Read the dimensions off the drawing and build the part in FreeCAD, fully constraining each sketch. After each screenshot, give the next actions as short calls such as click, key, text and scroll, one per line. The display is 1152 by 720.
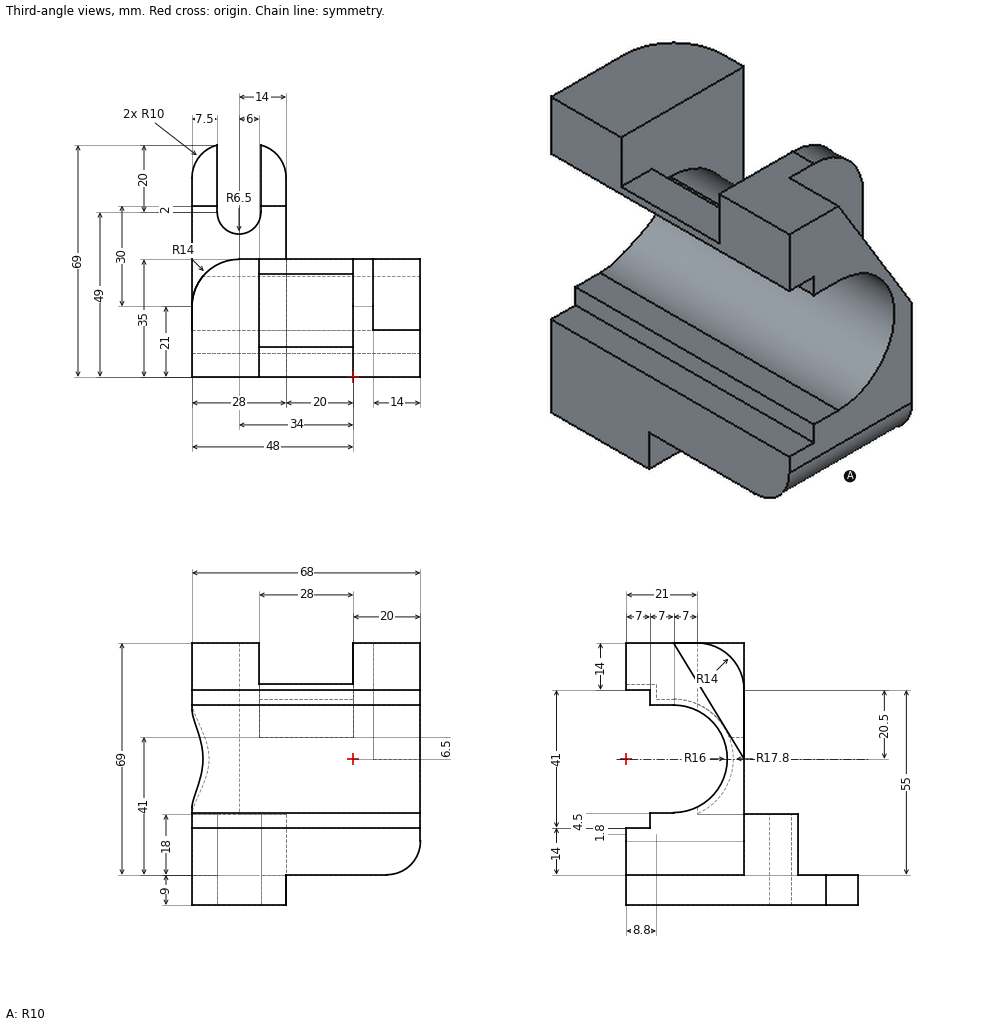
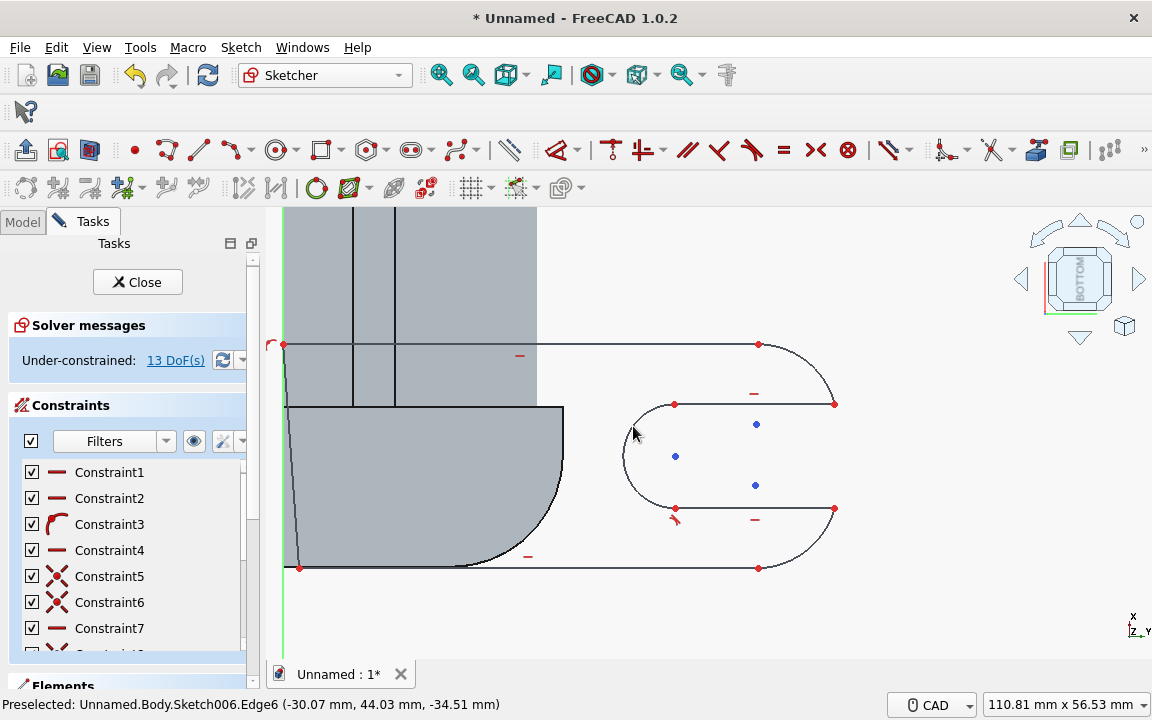
click(723, 404)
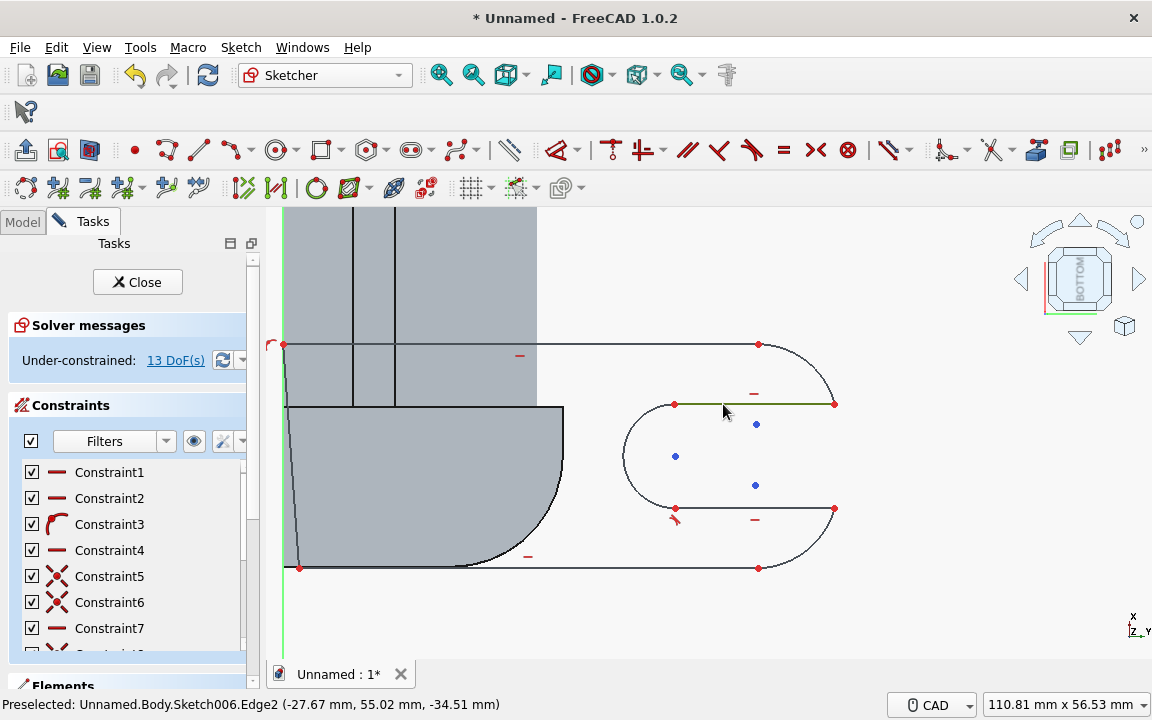
click(633, 426)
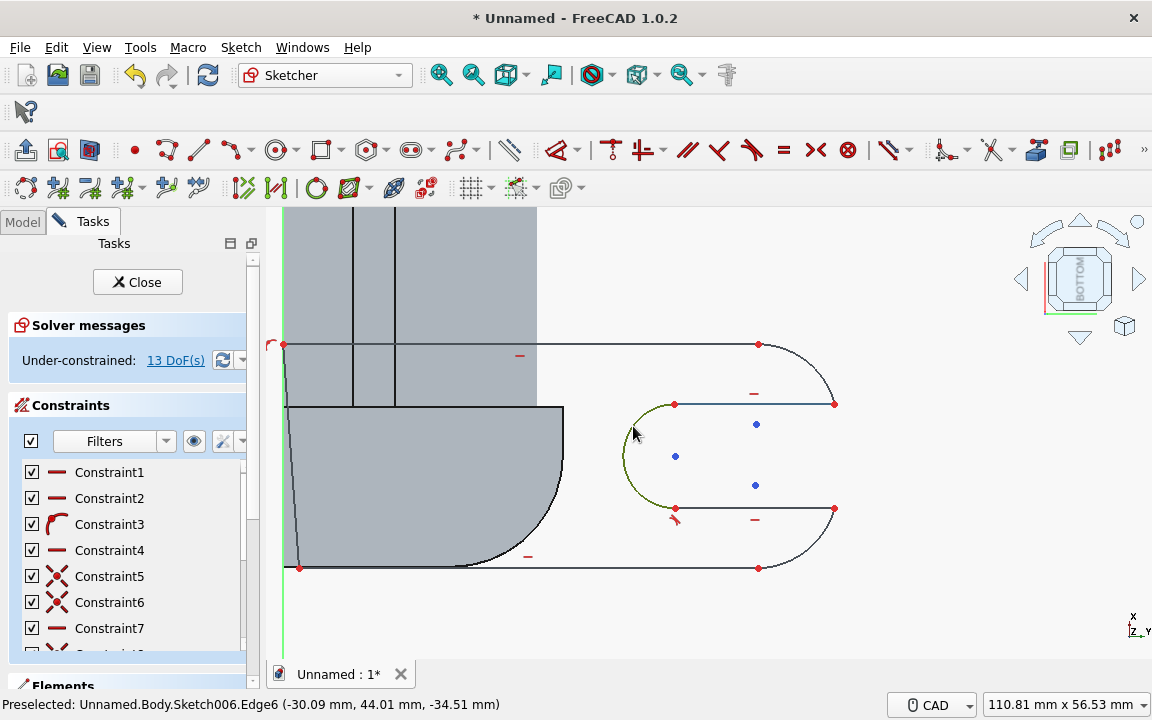
click(752, 150)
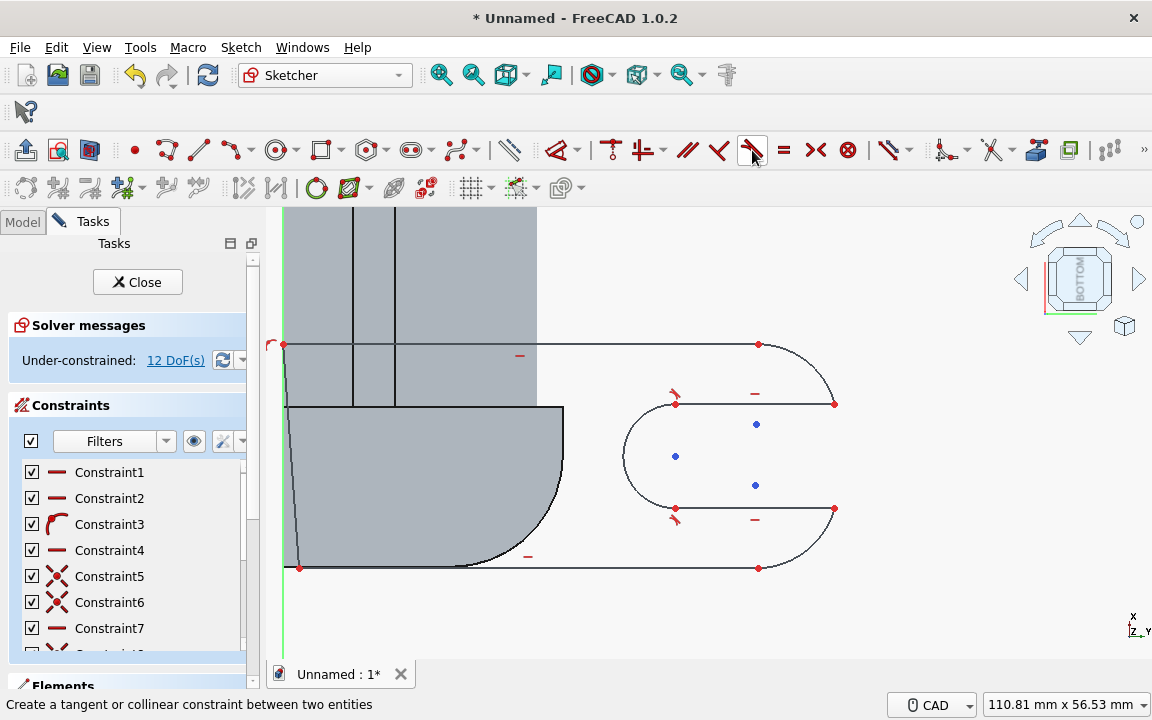
click(616, 344)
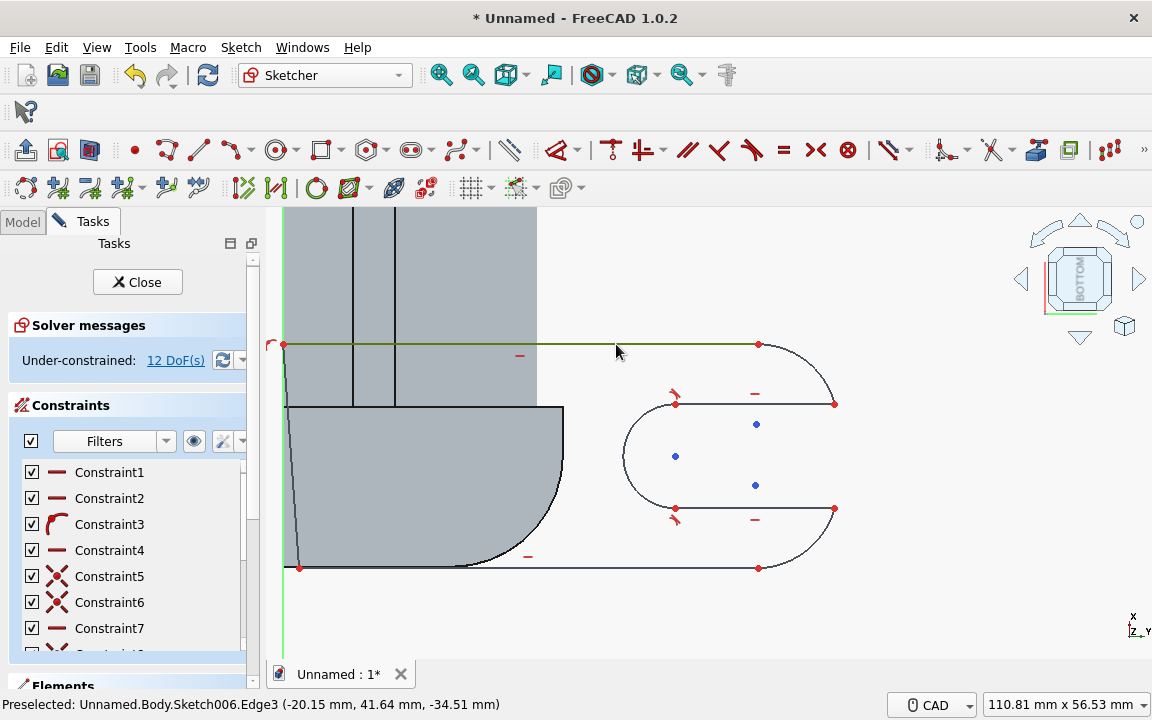
click(821, 376)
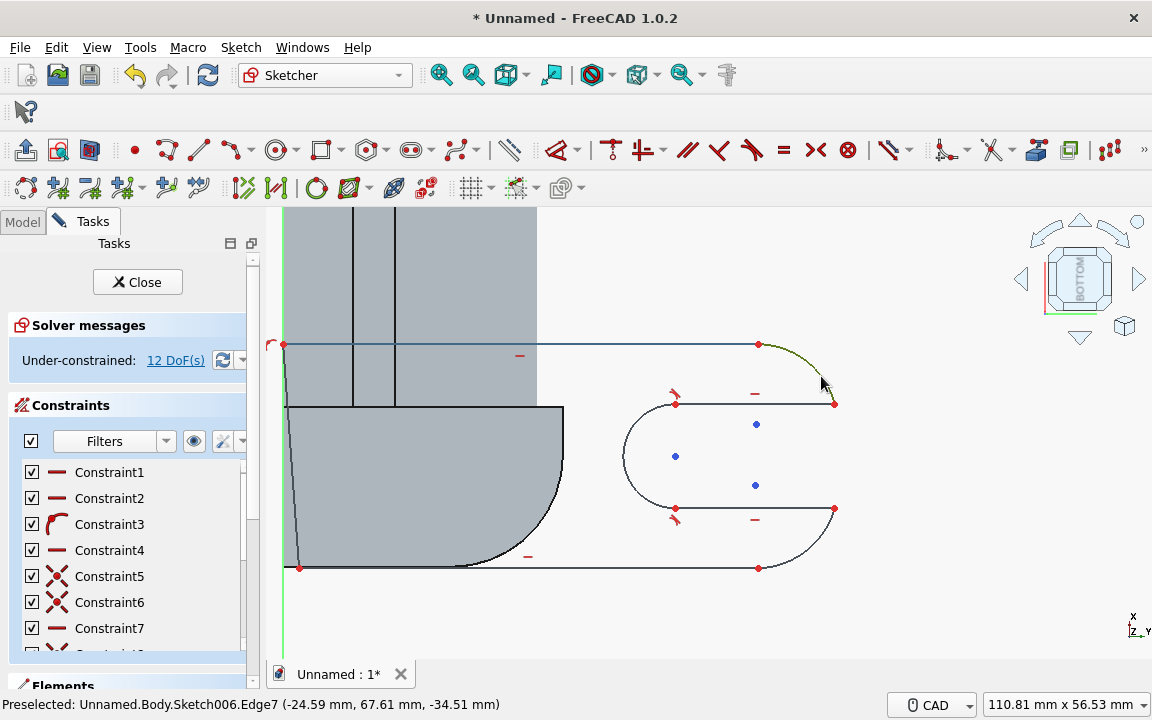
click(752, 150)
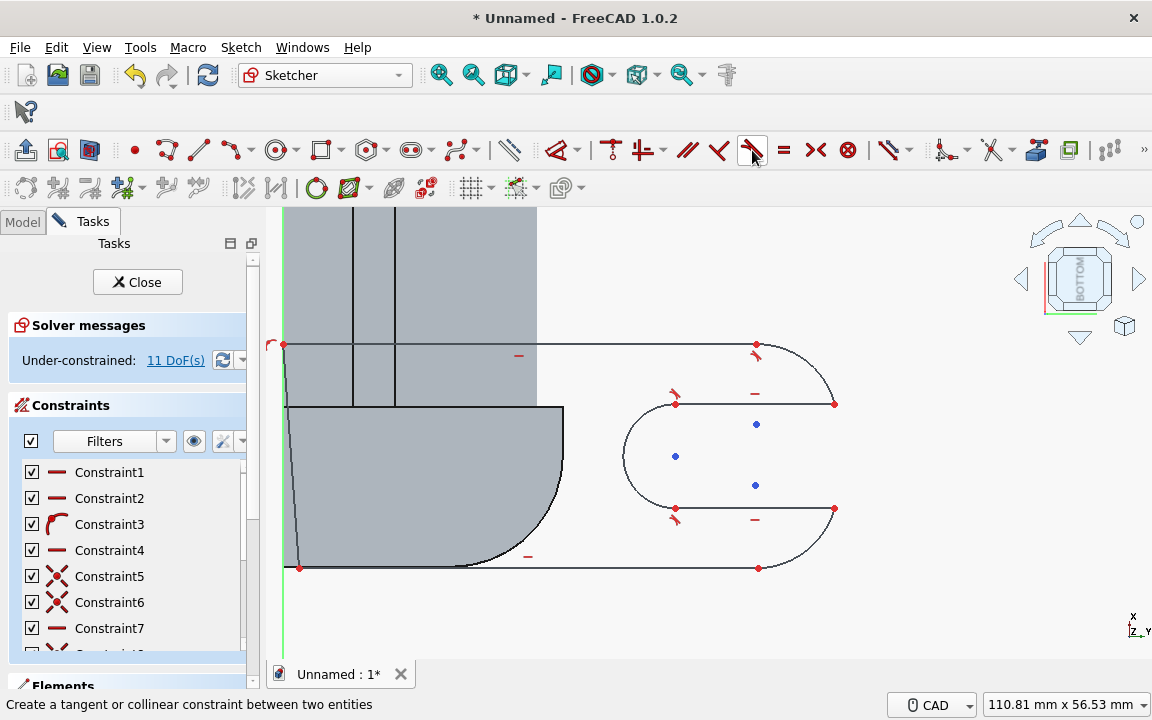
click(437, 568)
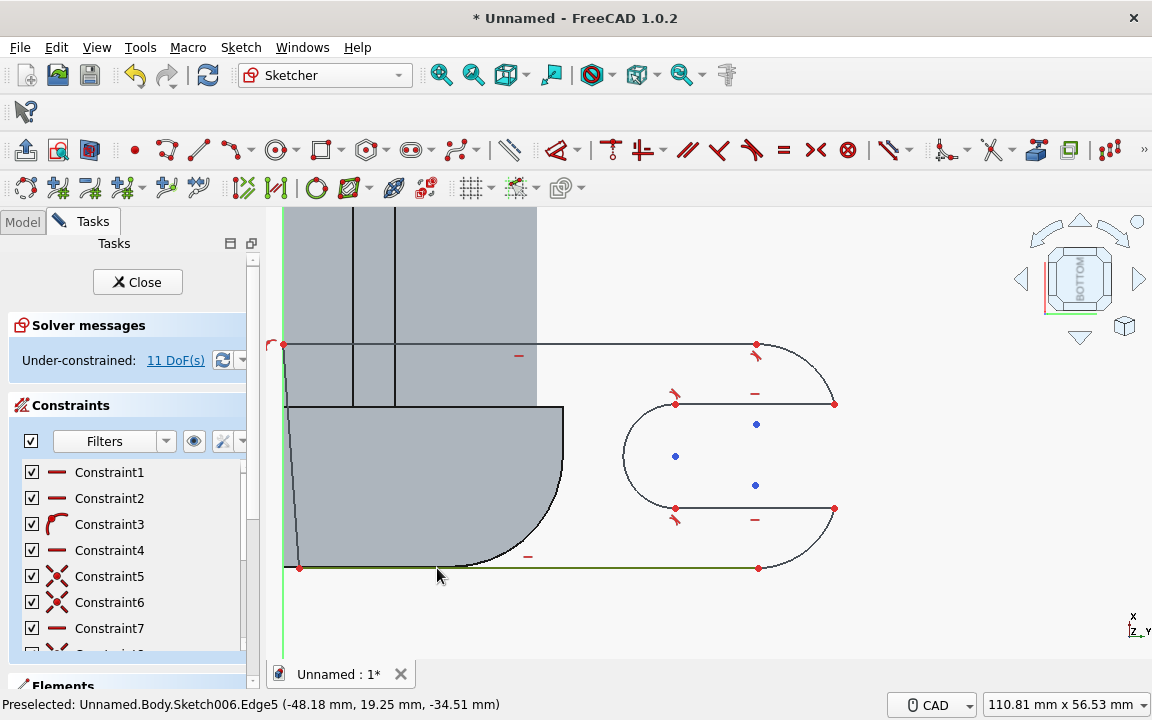
click(789, 561)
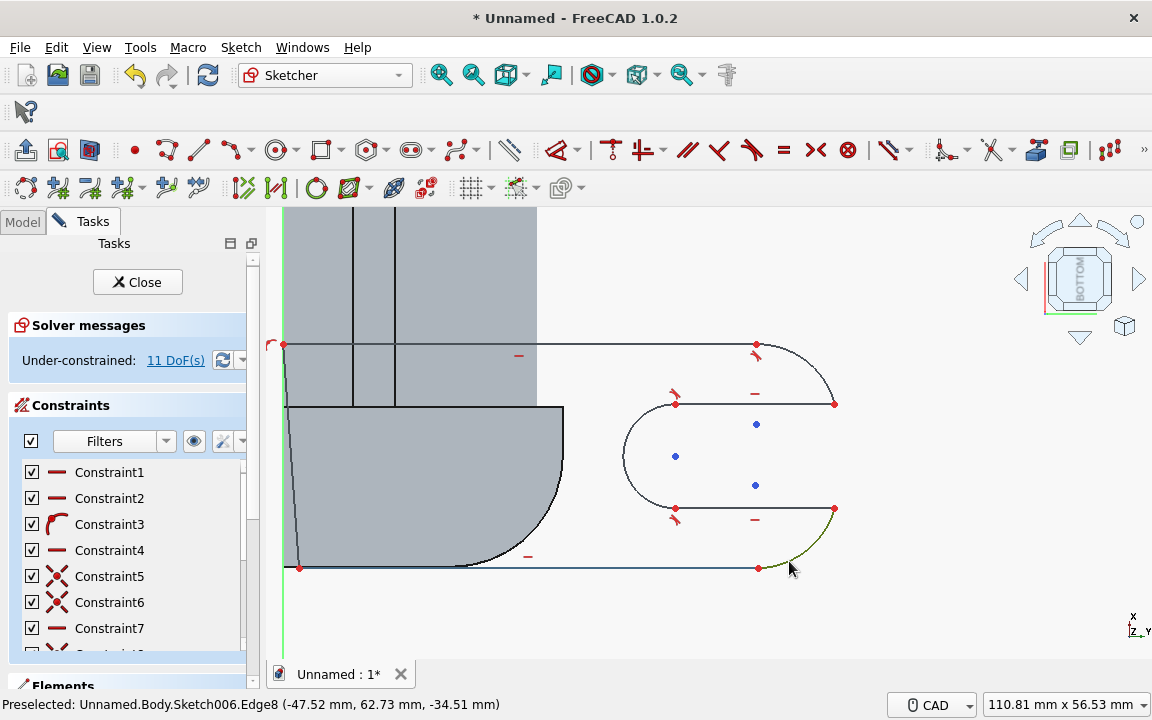
key(t)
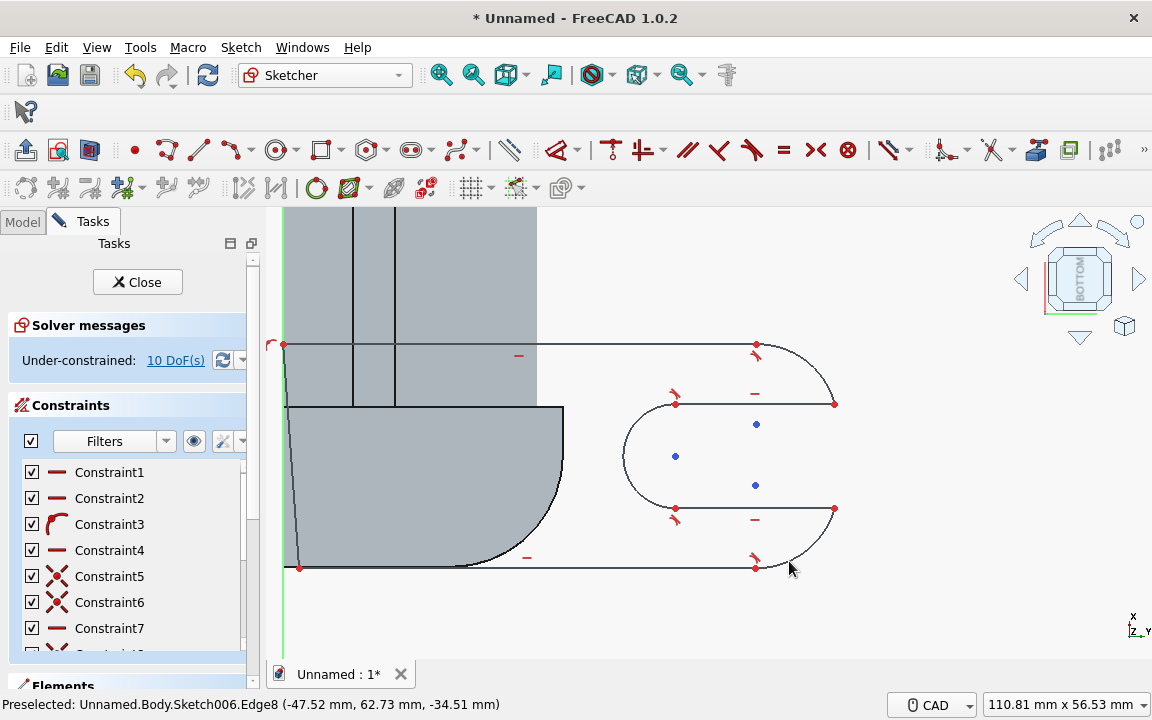
scroll(294, 501, up, 2)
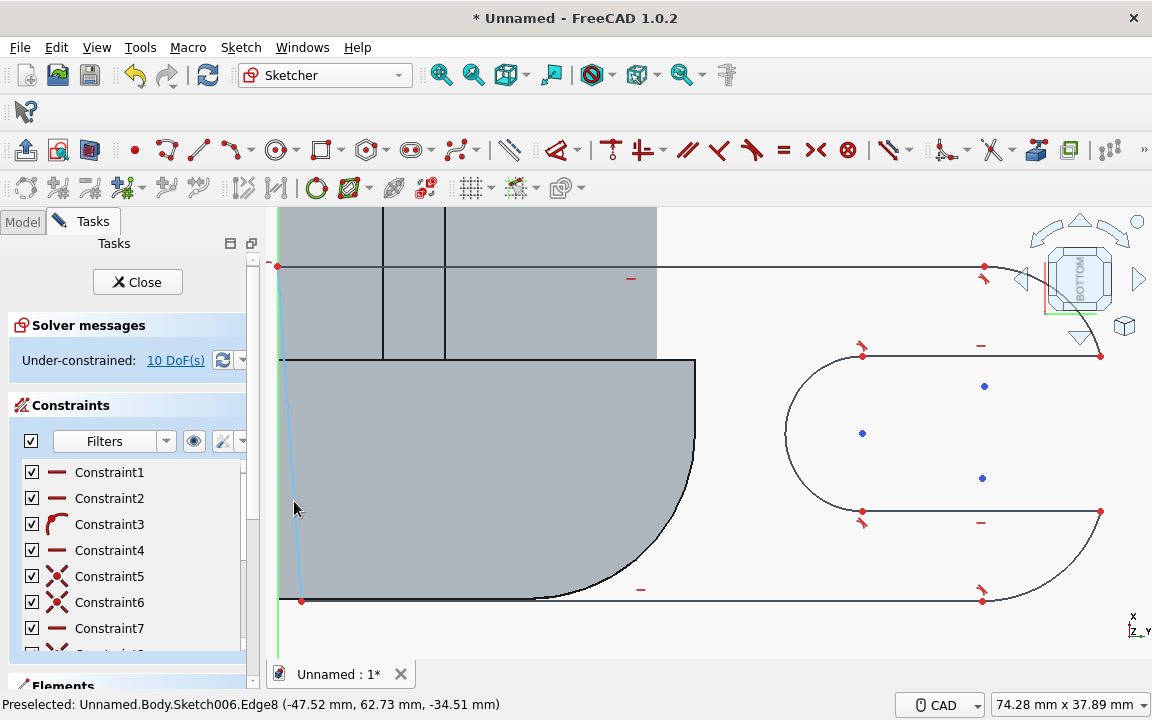
click(294, 501)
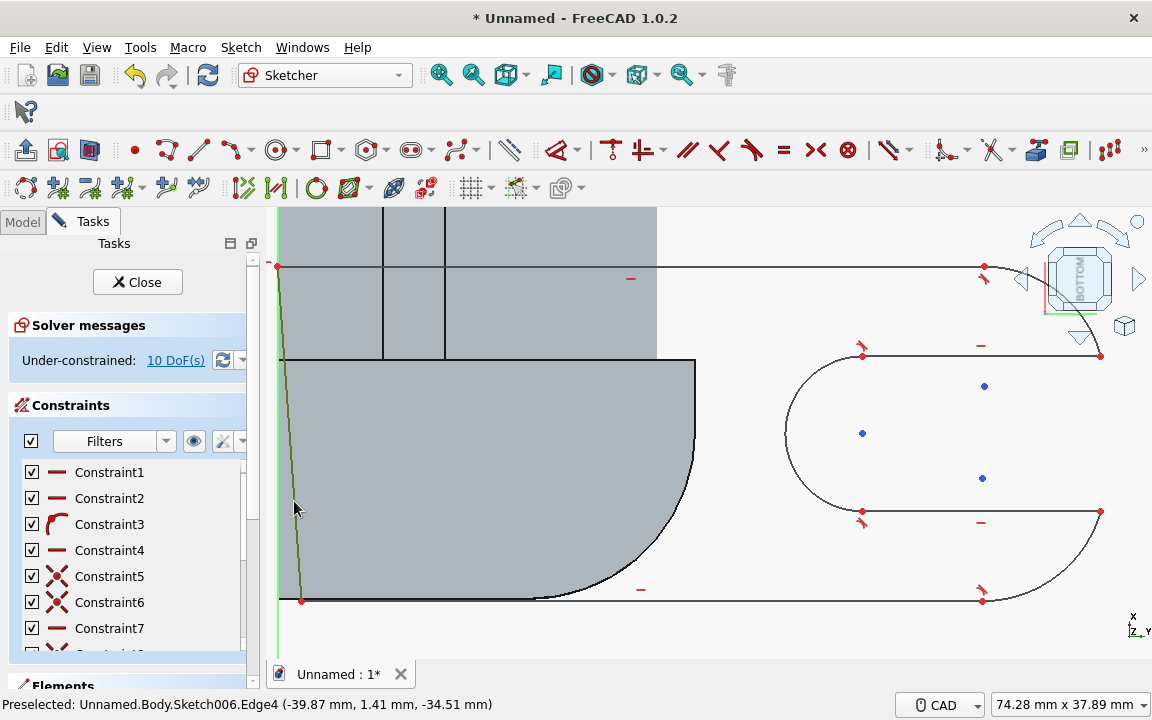
key(v)